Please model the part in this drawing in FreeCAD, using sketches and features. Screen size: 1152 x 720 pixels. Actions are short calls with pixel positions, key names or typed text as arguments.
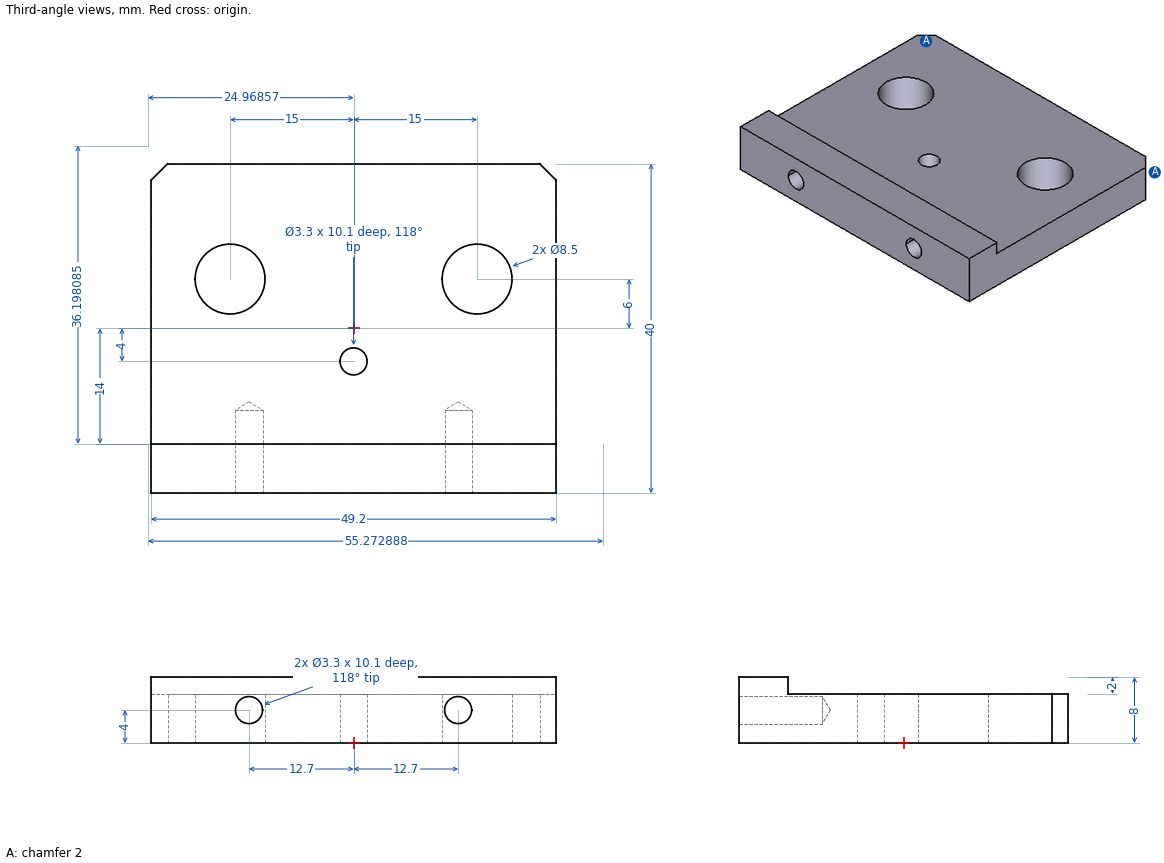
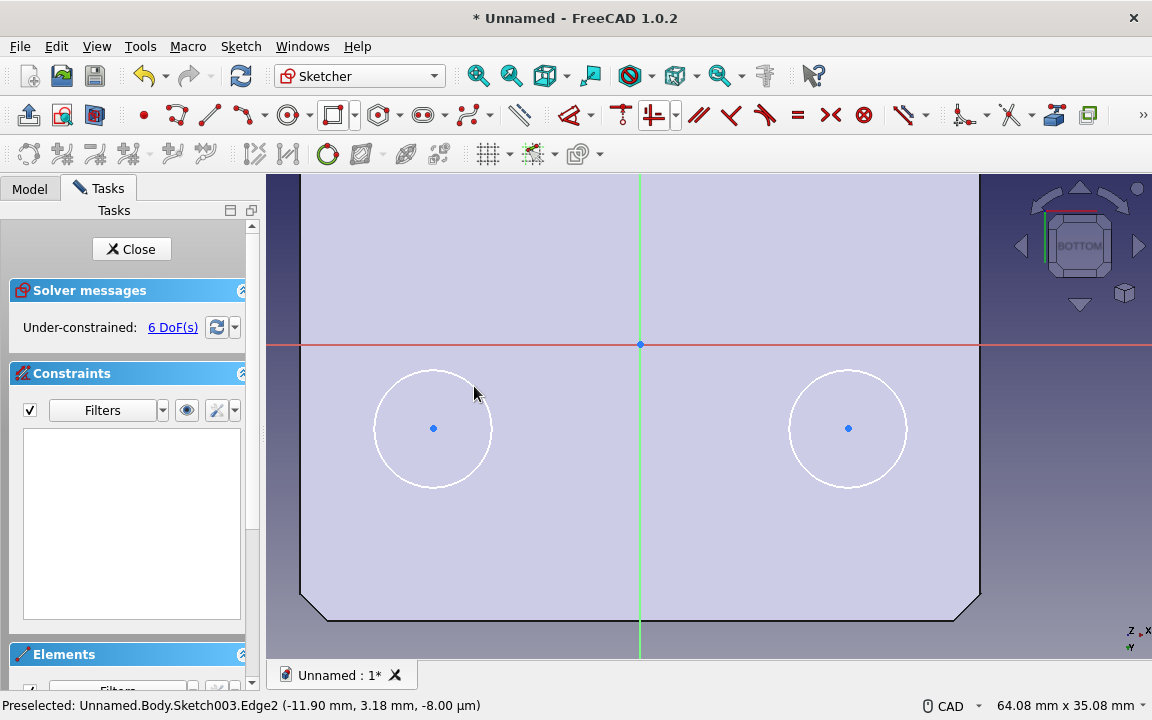
click(889, 387)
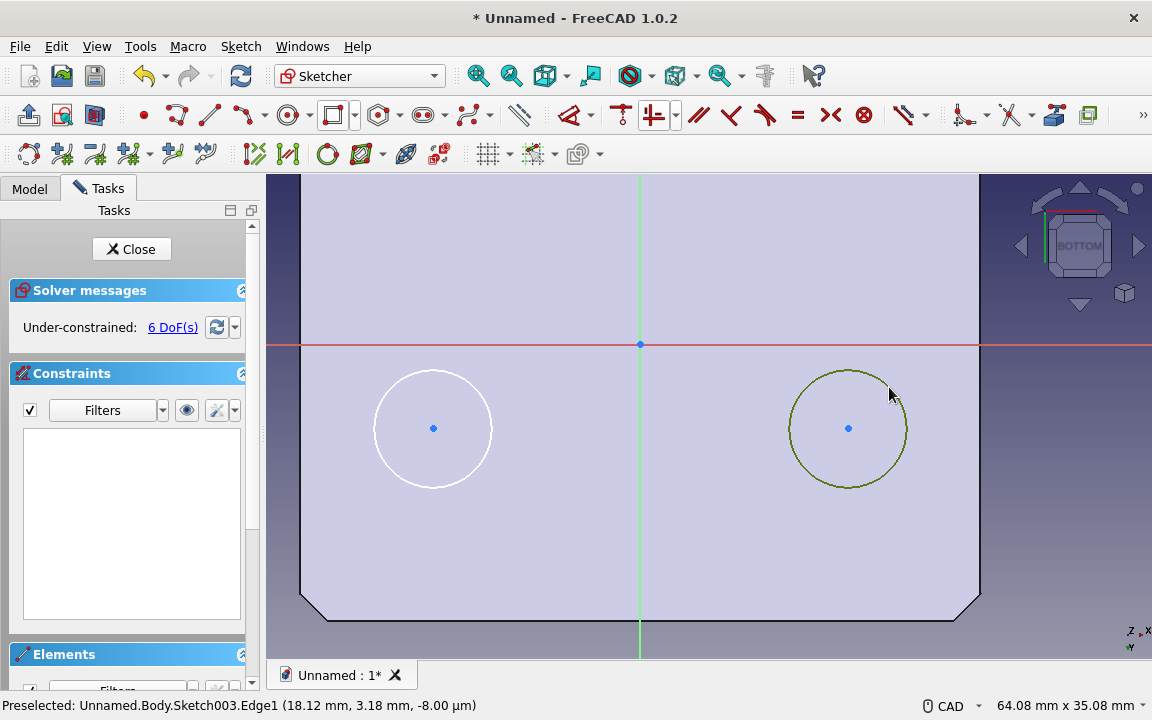
click(474, 387)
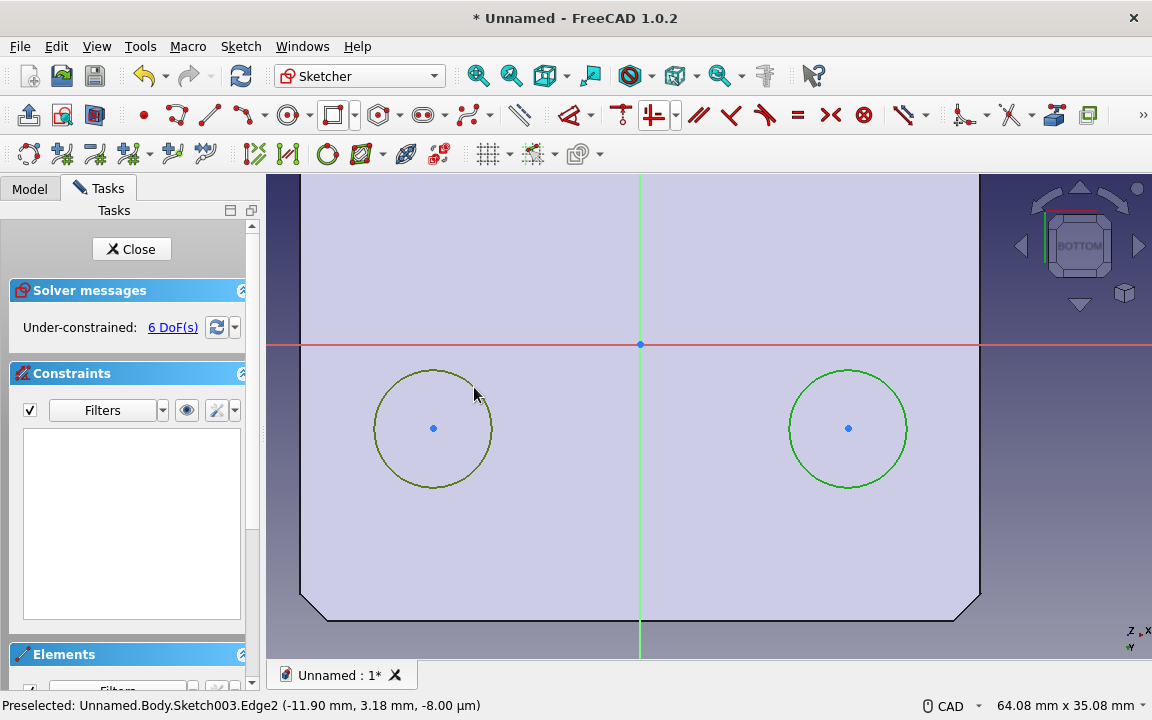
key(e)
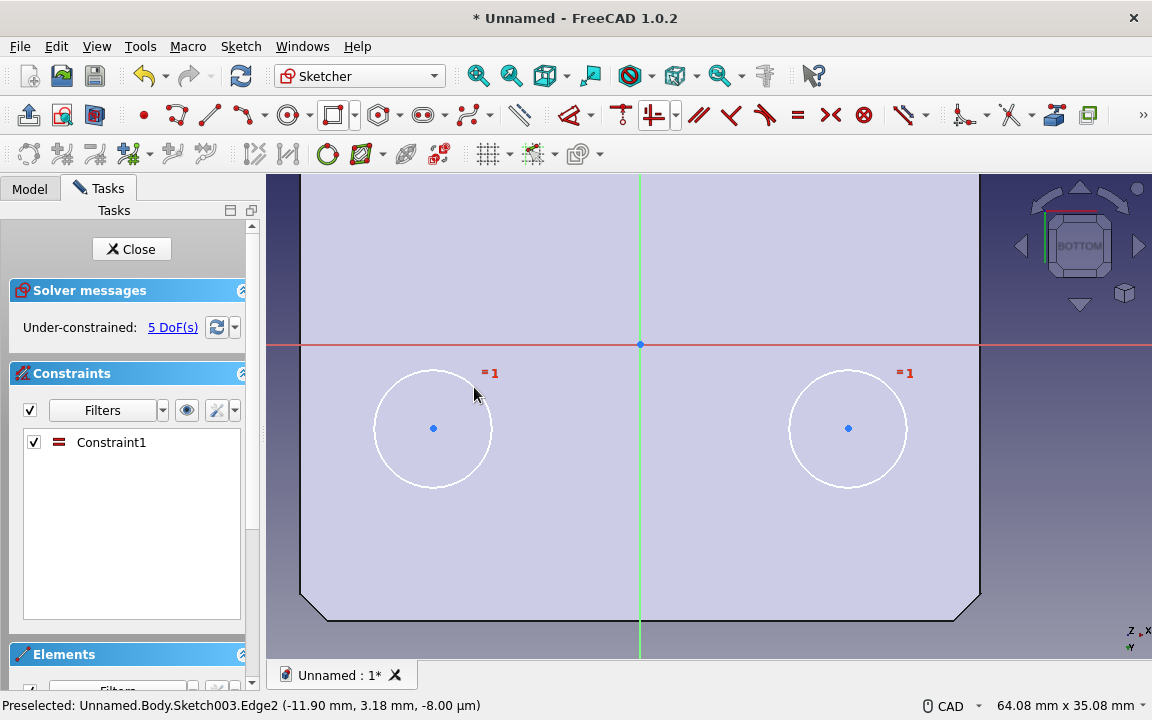
click(848, 429)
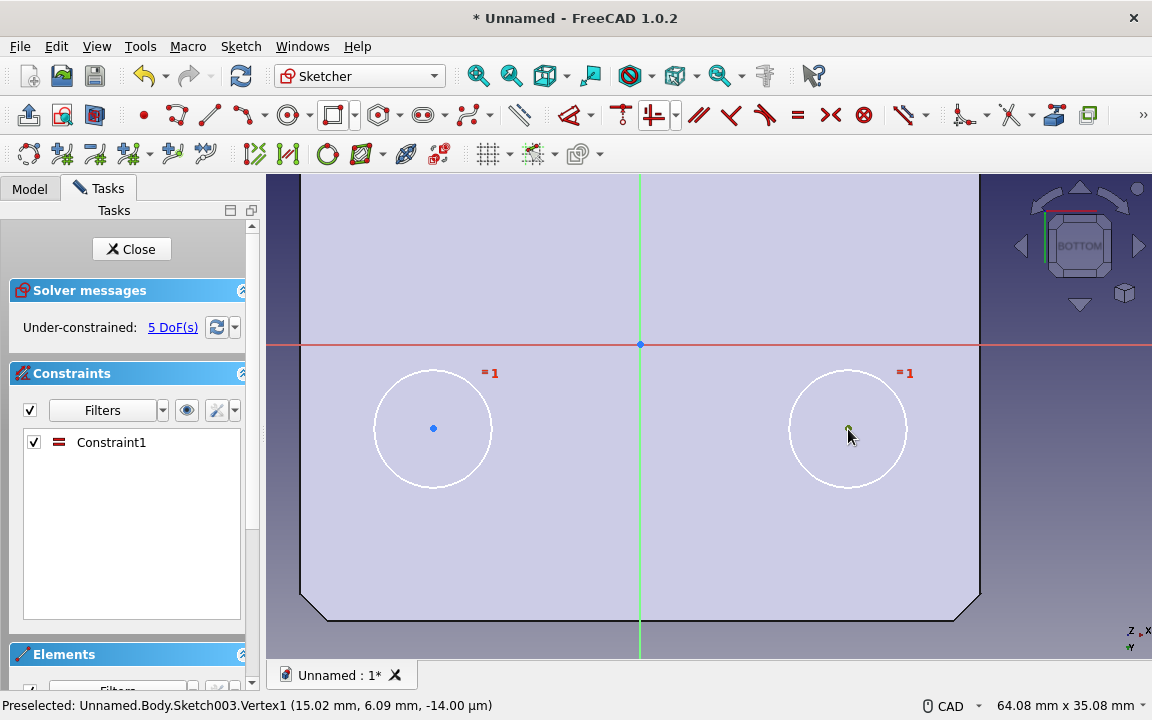
click(433, 429)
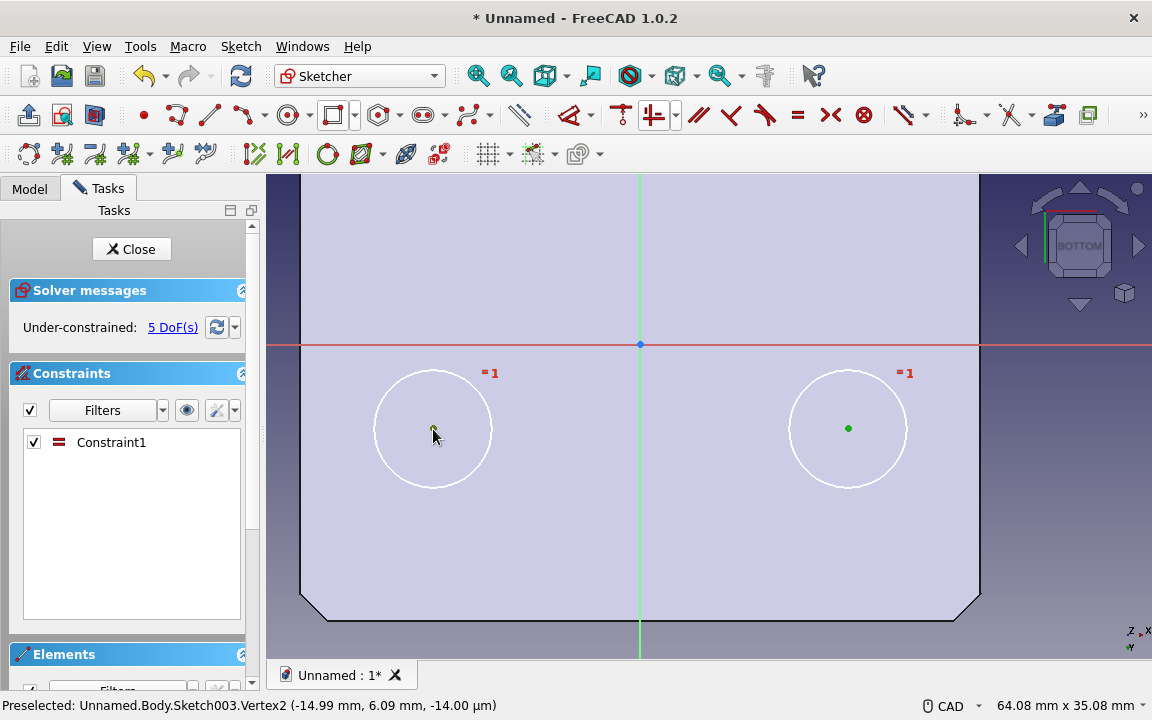
key(h)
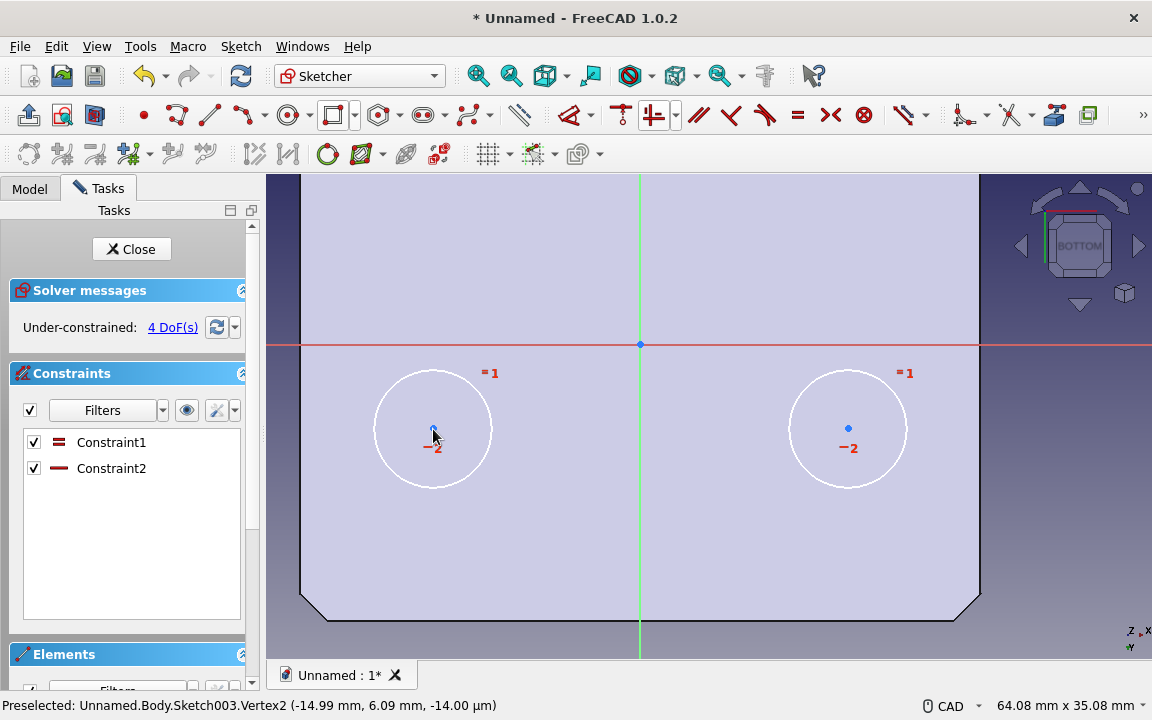
click(568, 116)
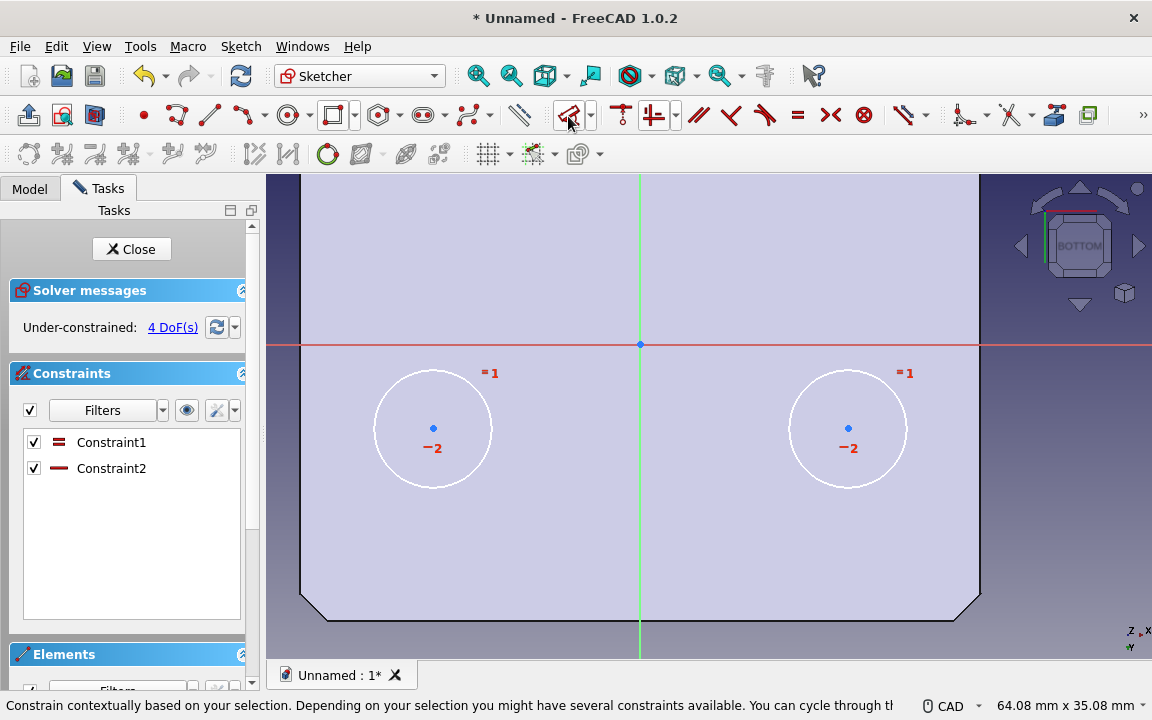
click(889, 387)
click(911, 364)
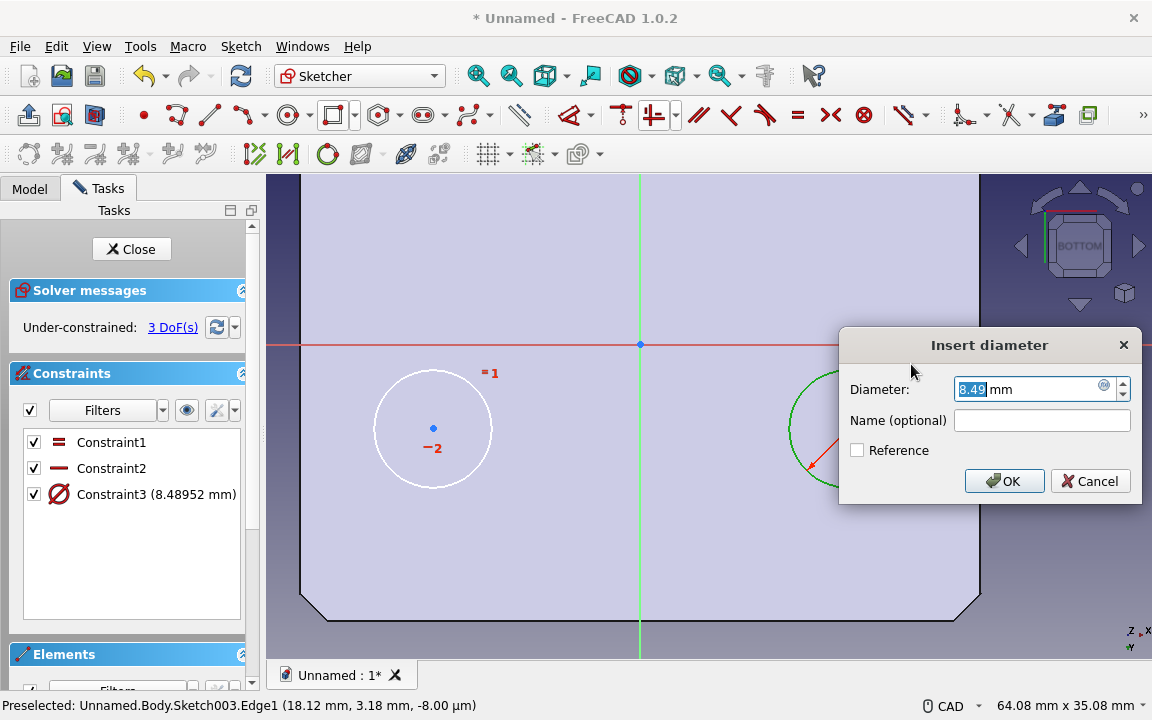
text(8.5)
key(Return)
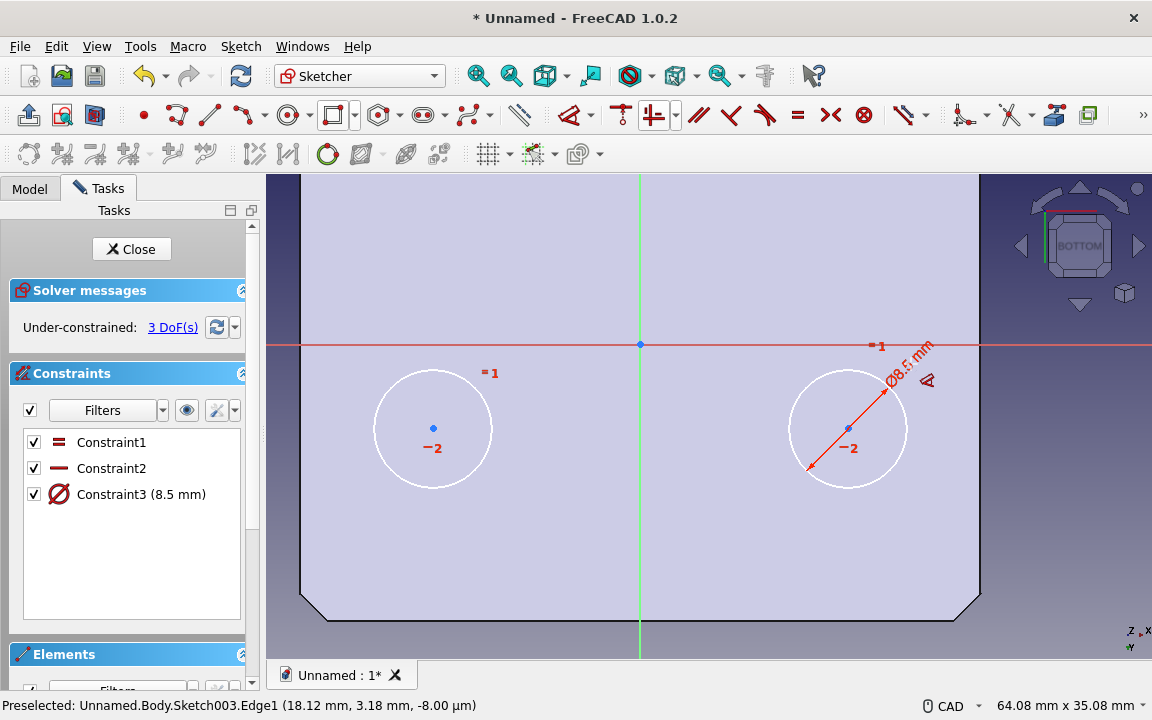
click(848, 429)
click(882, 406)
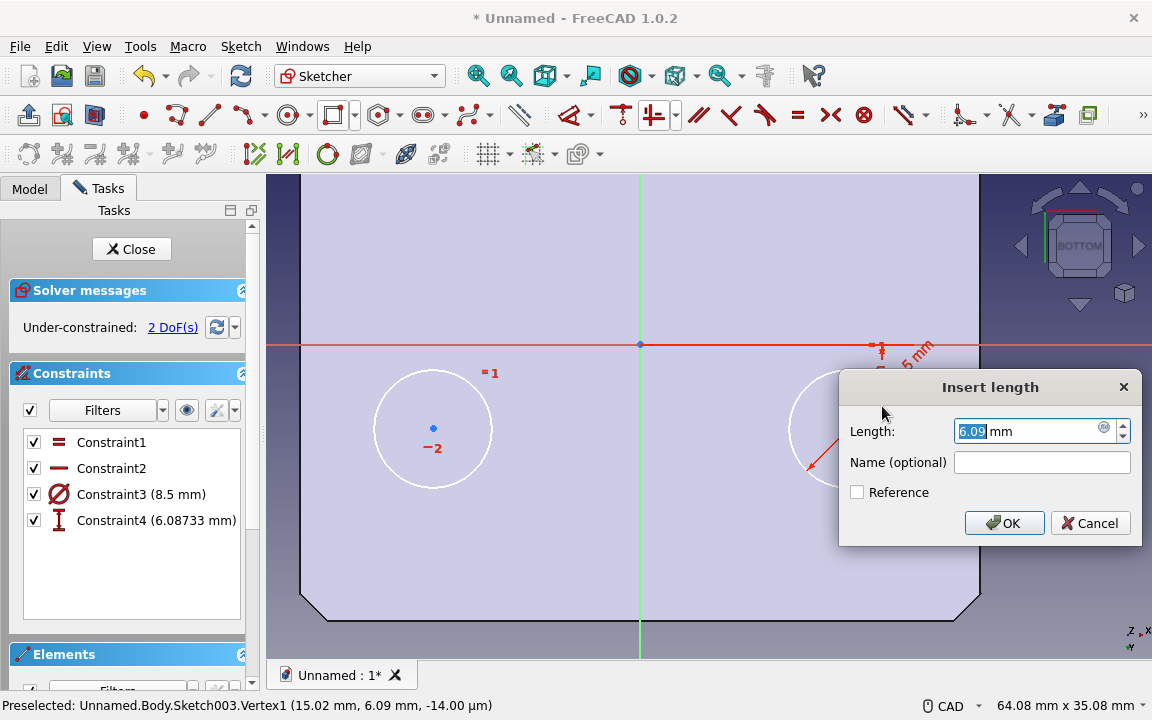
text(6)
key(Return)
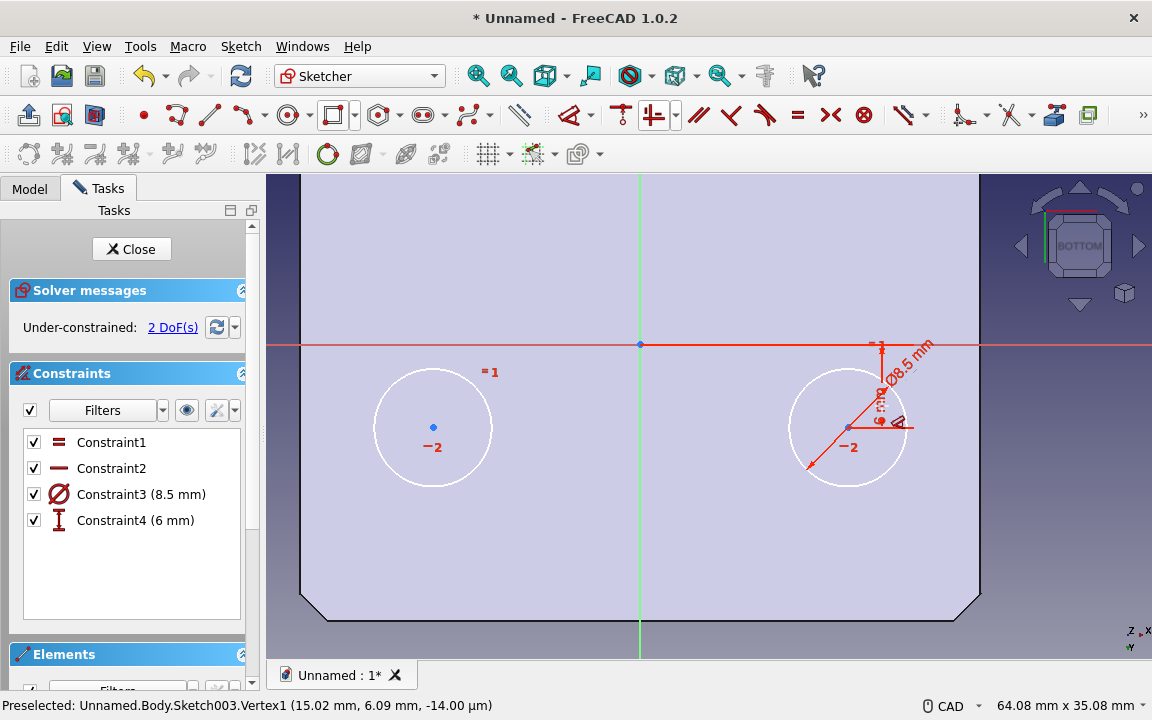
click(848, 428)
click(744, 311)